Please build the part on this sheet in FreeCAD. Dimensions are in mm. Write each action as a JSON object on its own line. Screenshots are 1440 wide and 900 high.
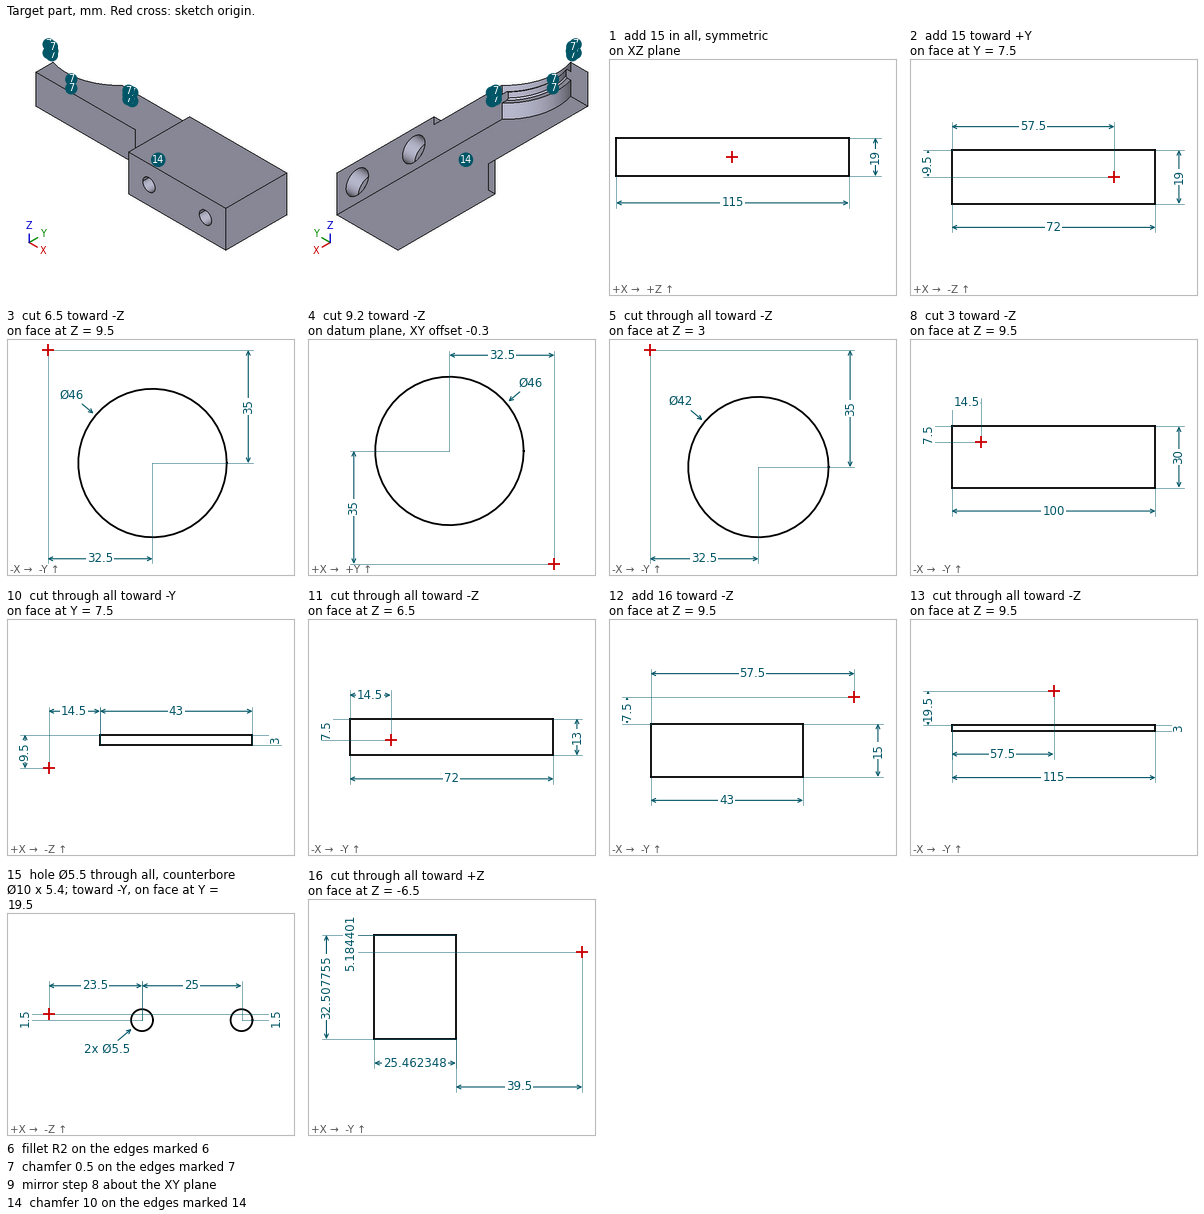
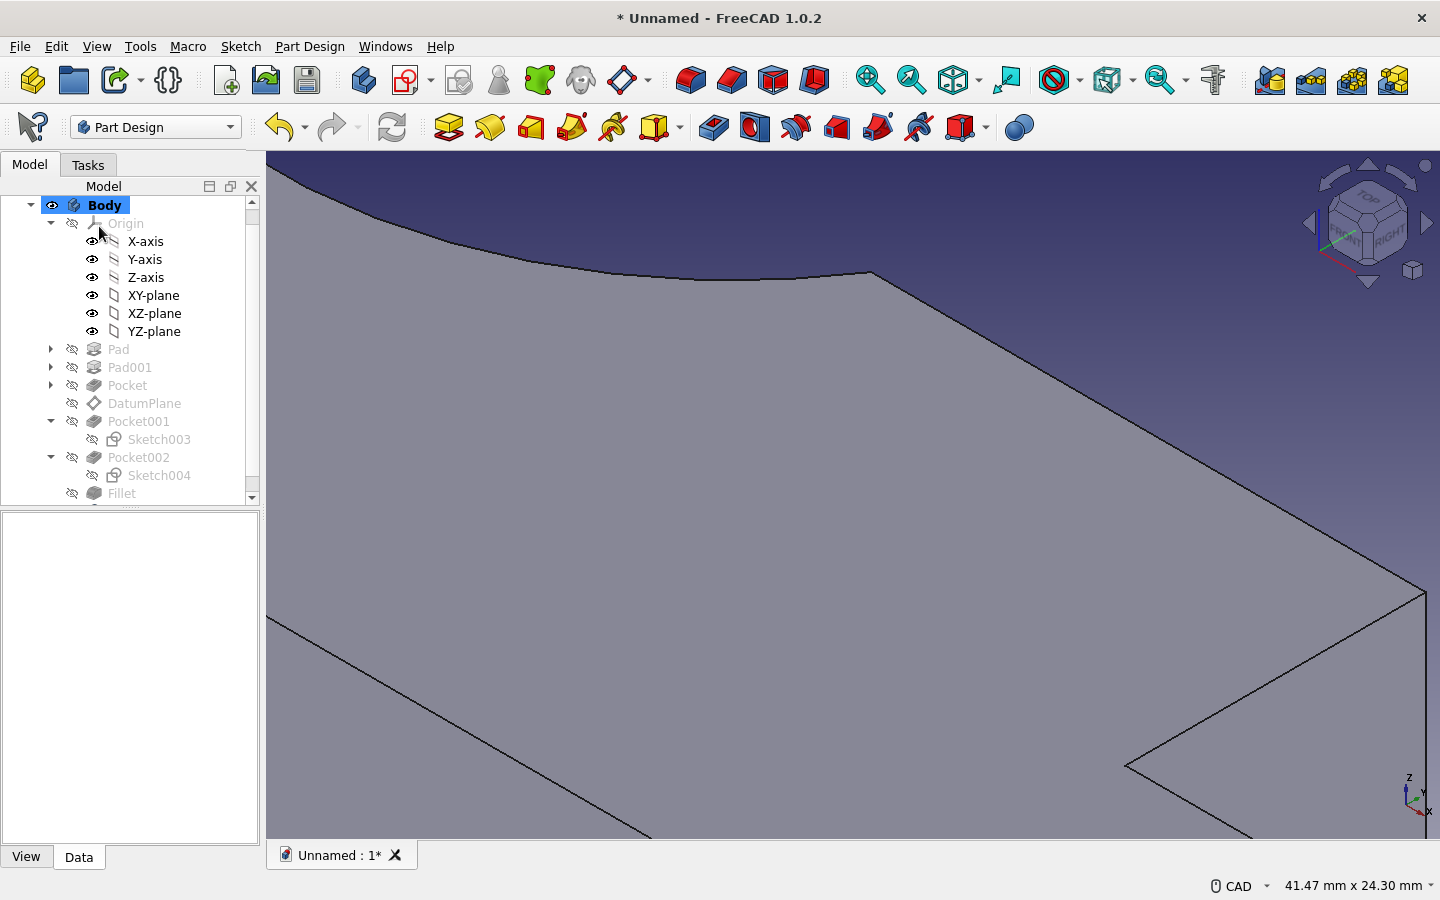
{"action": "left_click", "coordinate": [871, 80]}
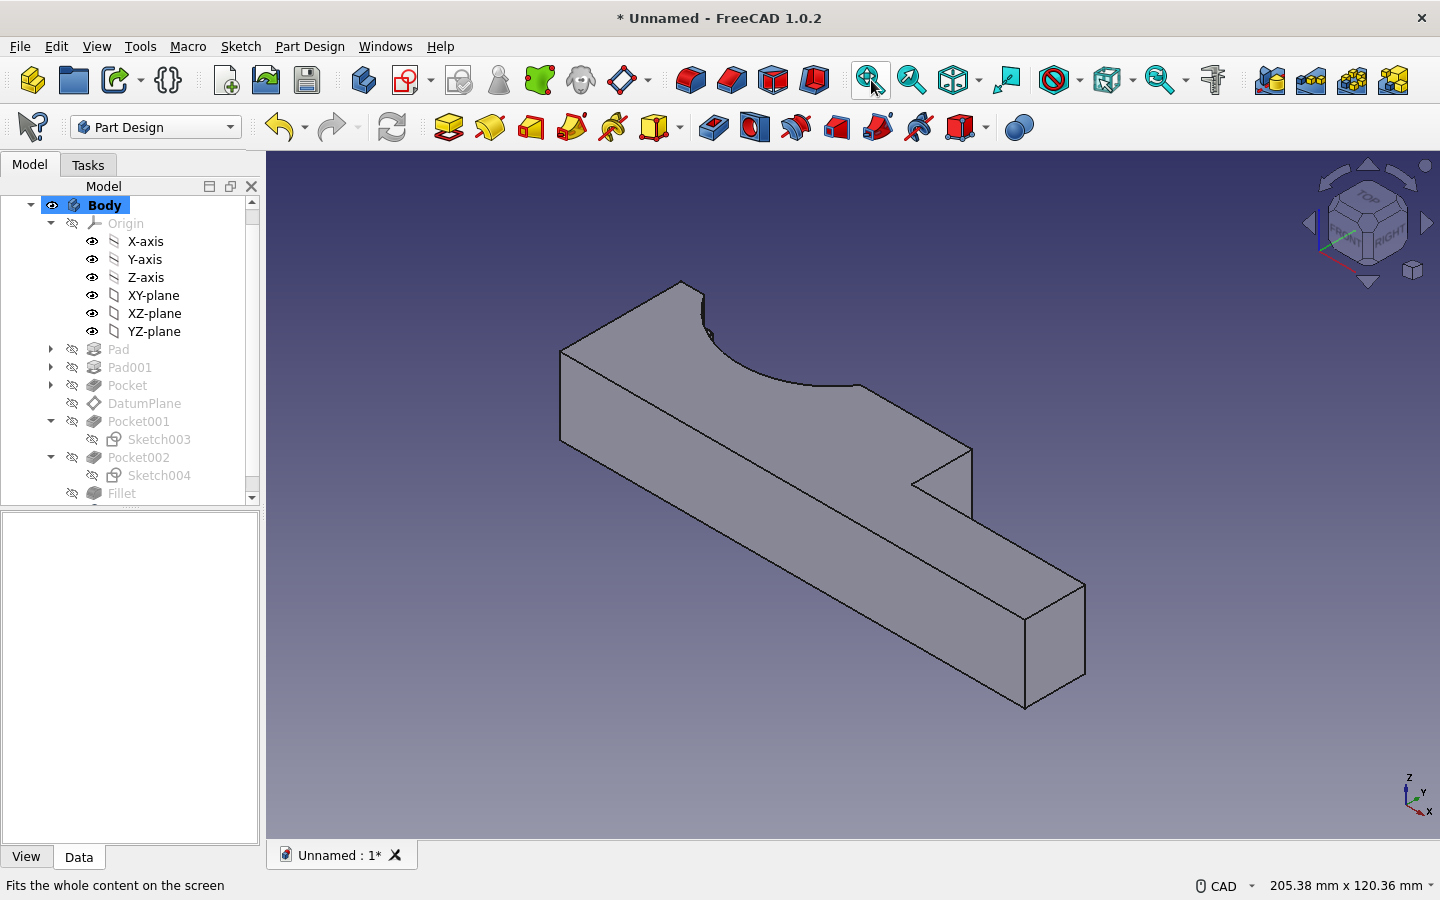
{"action": "left_click", "coordinate": [853, 450]}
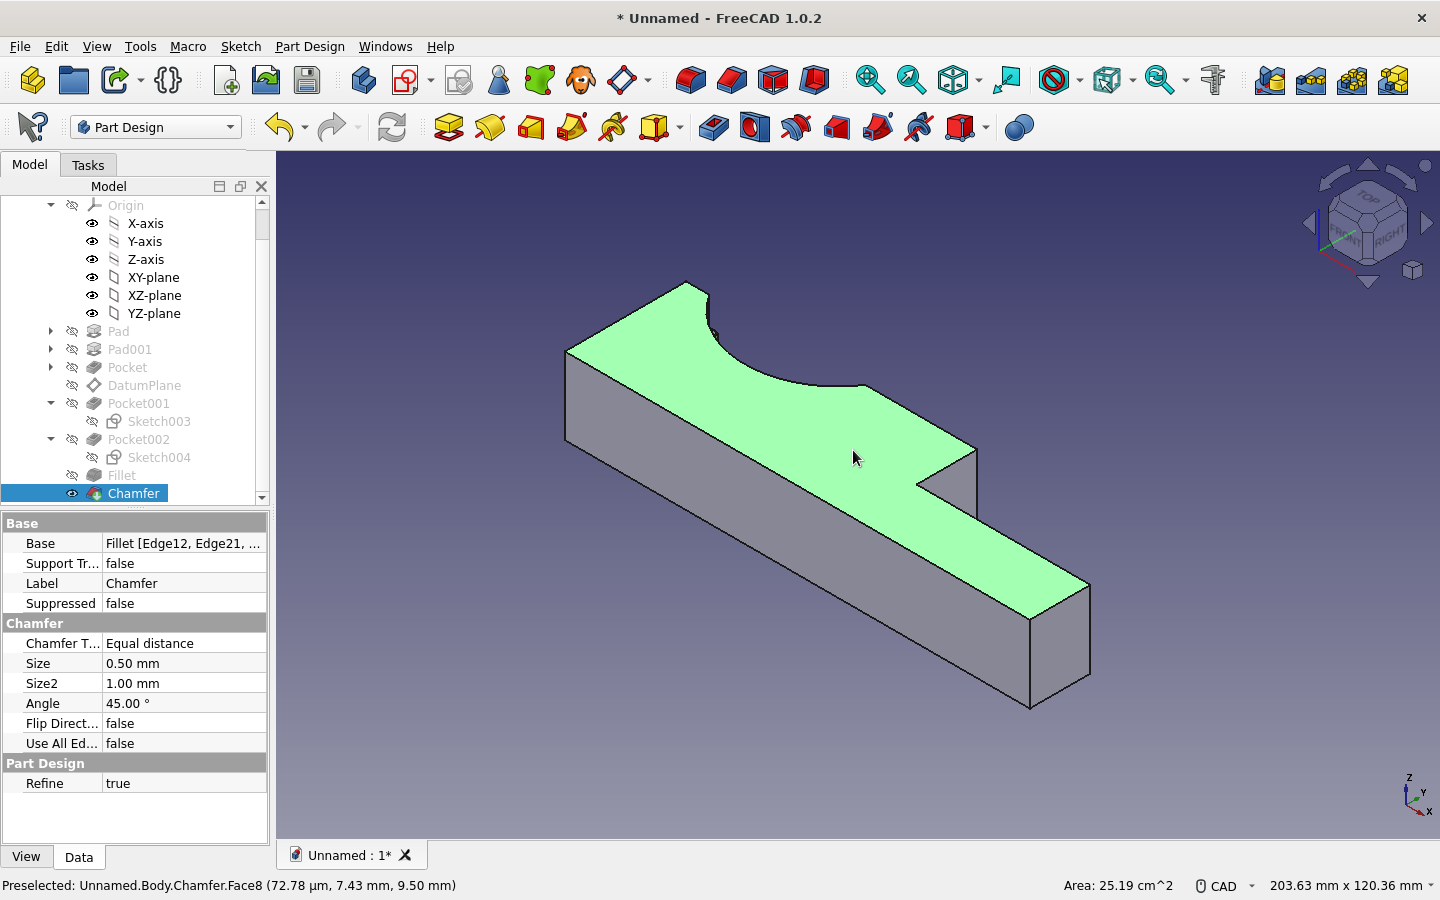
{"action": "left_click", "coordinate": [404, 80]}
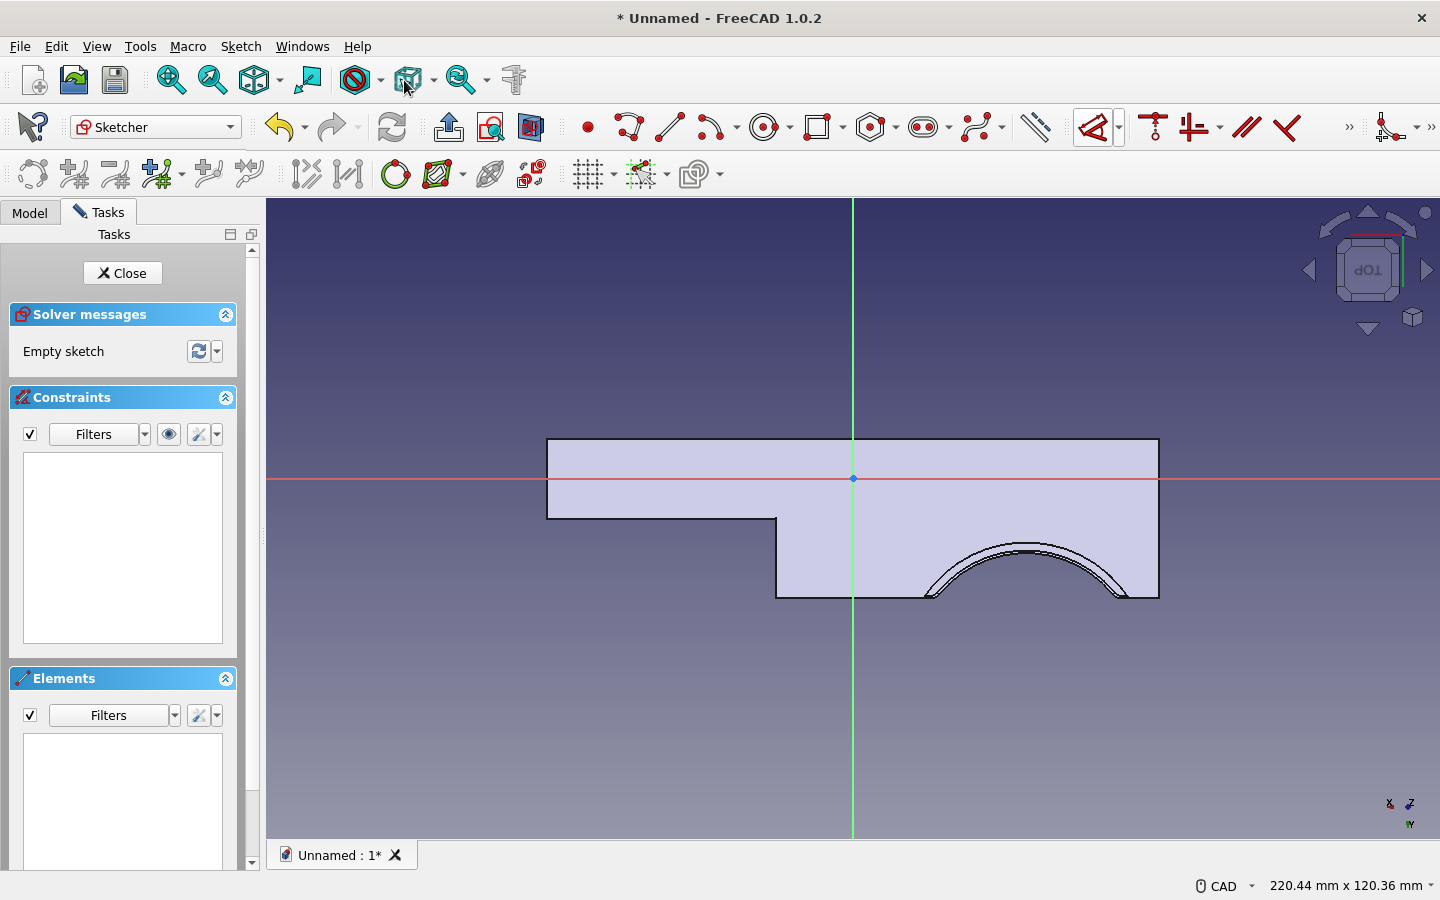
{"action": "scroll", "coordinate": [294, 519], "scroll_direction": "down", "scroll_amount": 1}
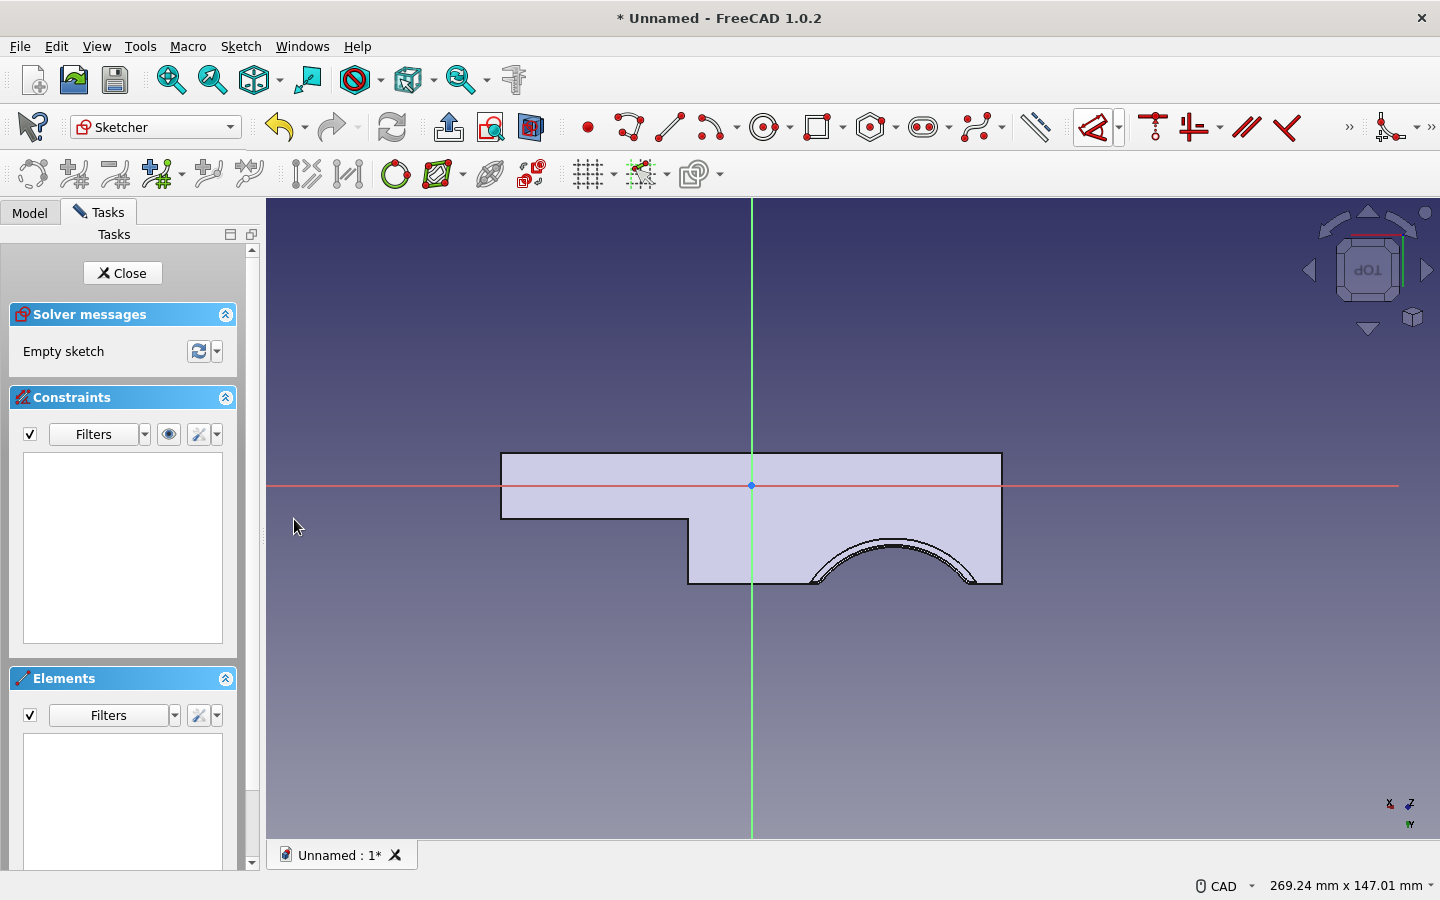
{"action": "scroll", "coordinate": [1154, 519], "scroll_direction": "up", "scroll_amount": 2}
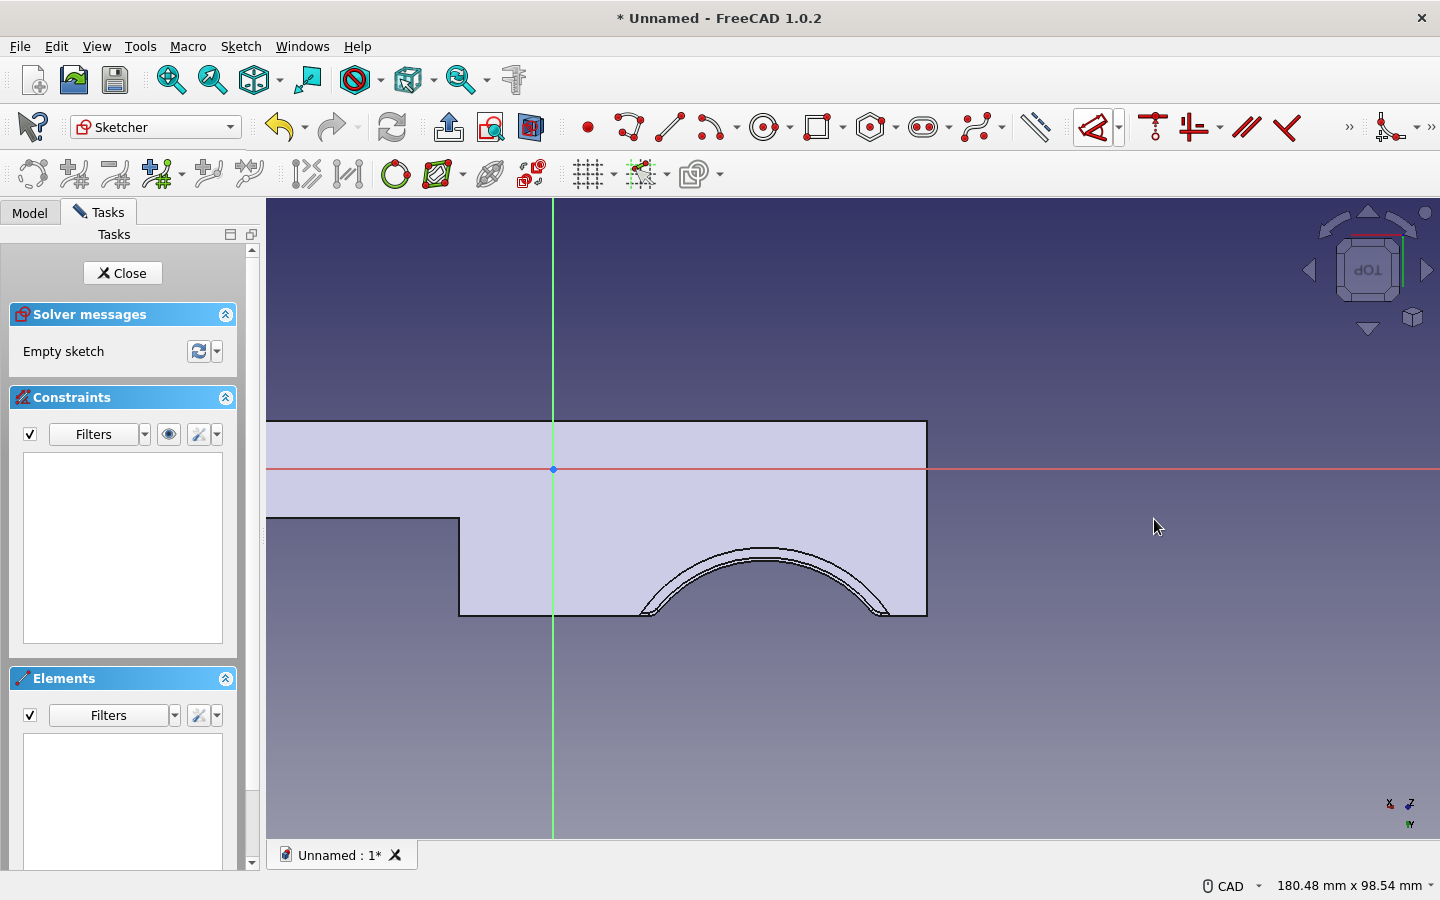
{"action": "left_click", "coordinate": [816, 128]}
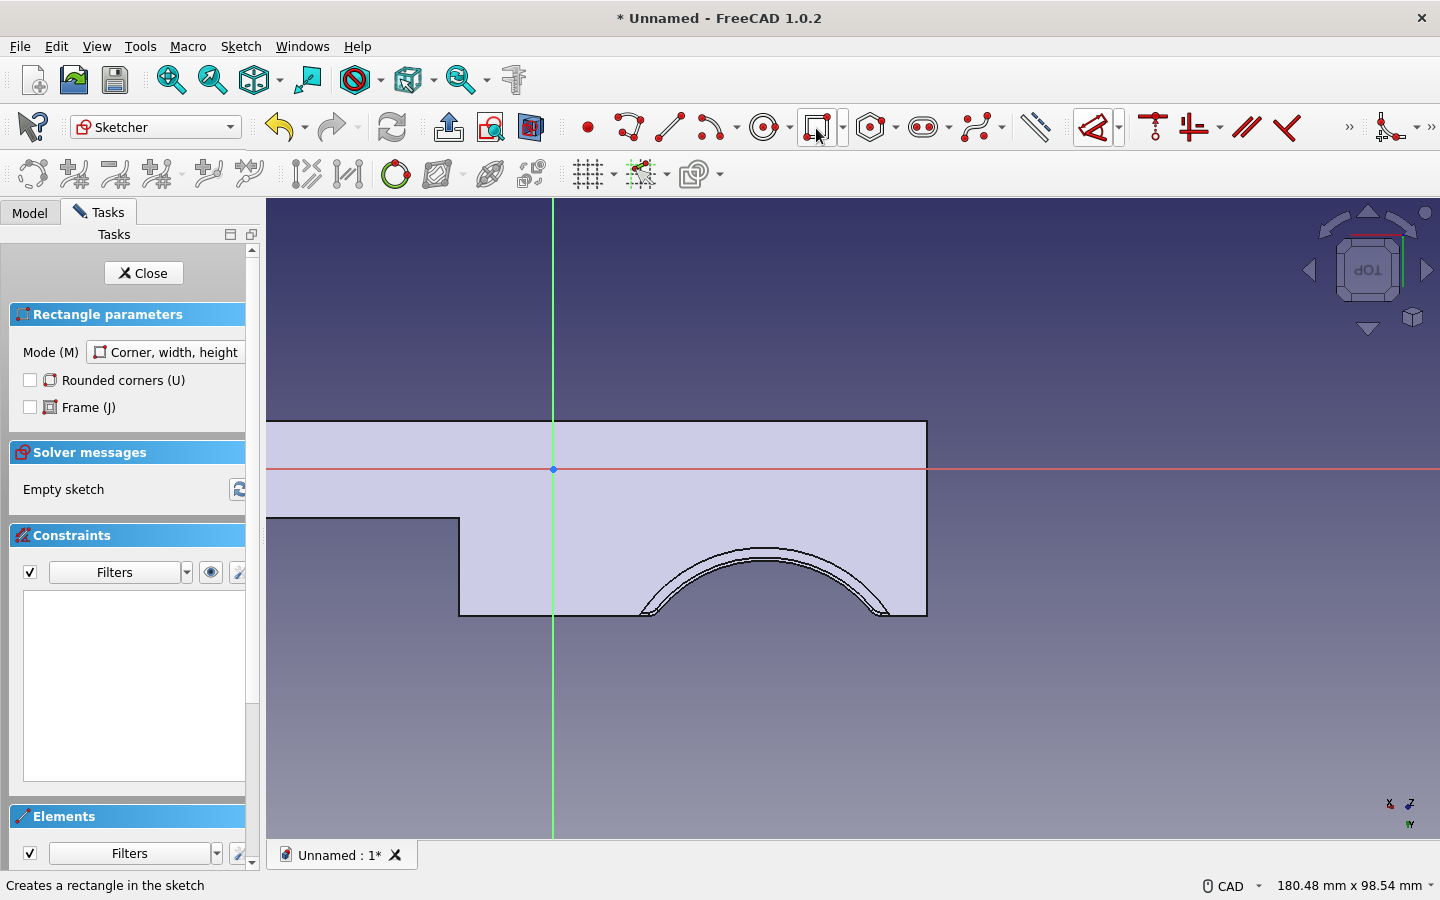
{"action": "left_click", "coordinate": [459, 421]}
{"action": "mouse_move", "coordinate": [1110, 616]}